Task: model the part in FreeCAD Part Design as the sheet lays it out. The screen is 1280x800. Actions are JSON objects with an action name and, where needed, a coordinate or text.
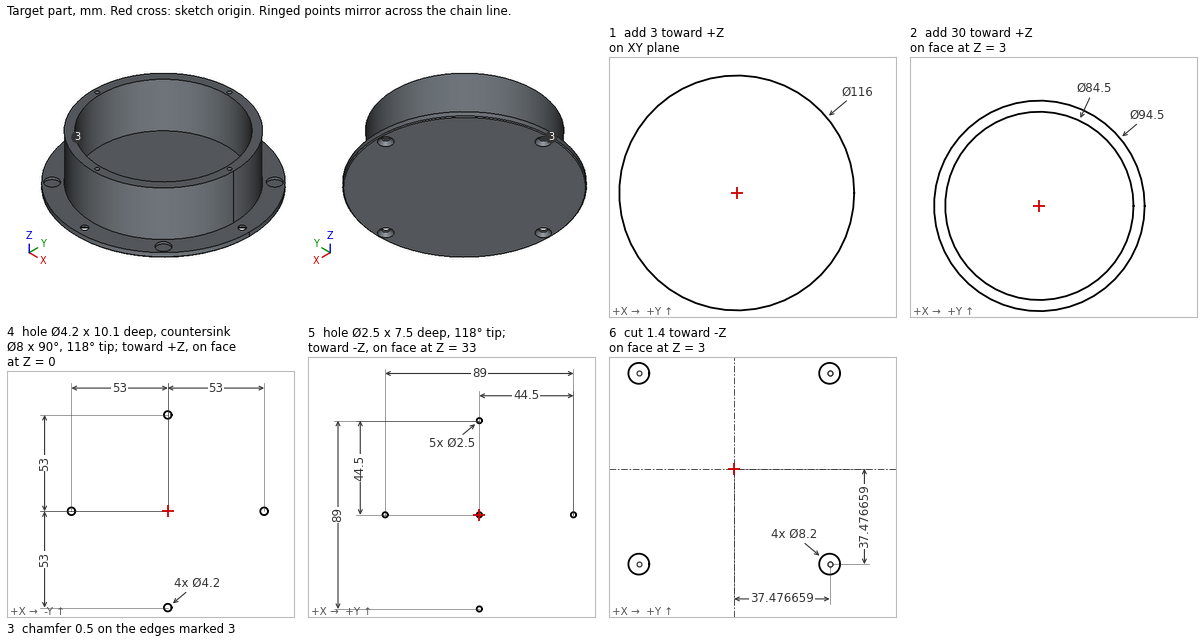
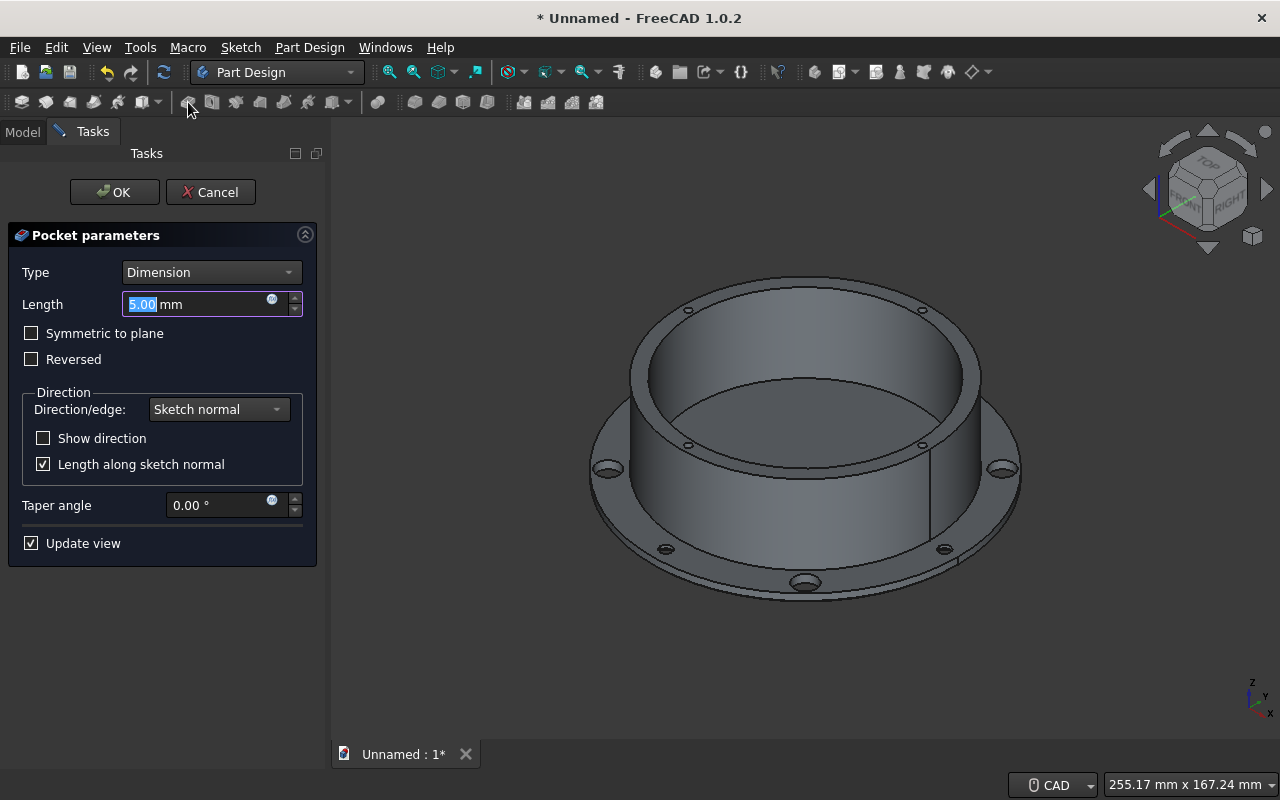
{"action": "type", "text": "1.4"}
{"action": "key", "text": "Tab"}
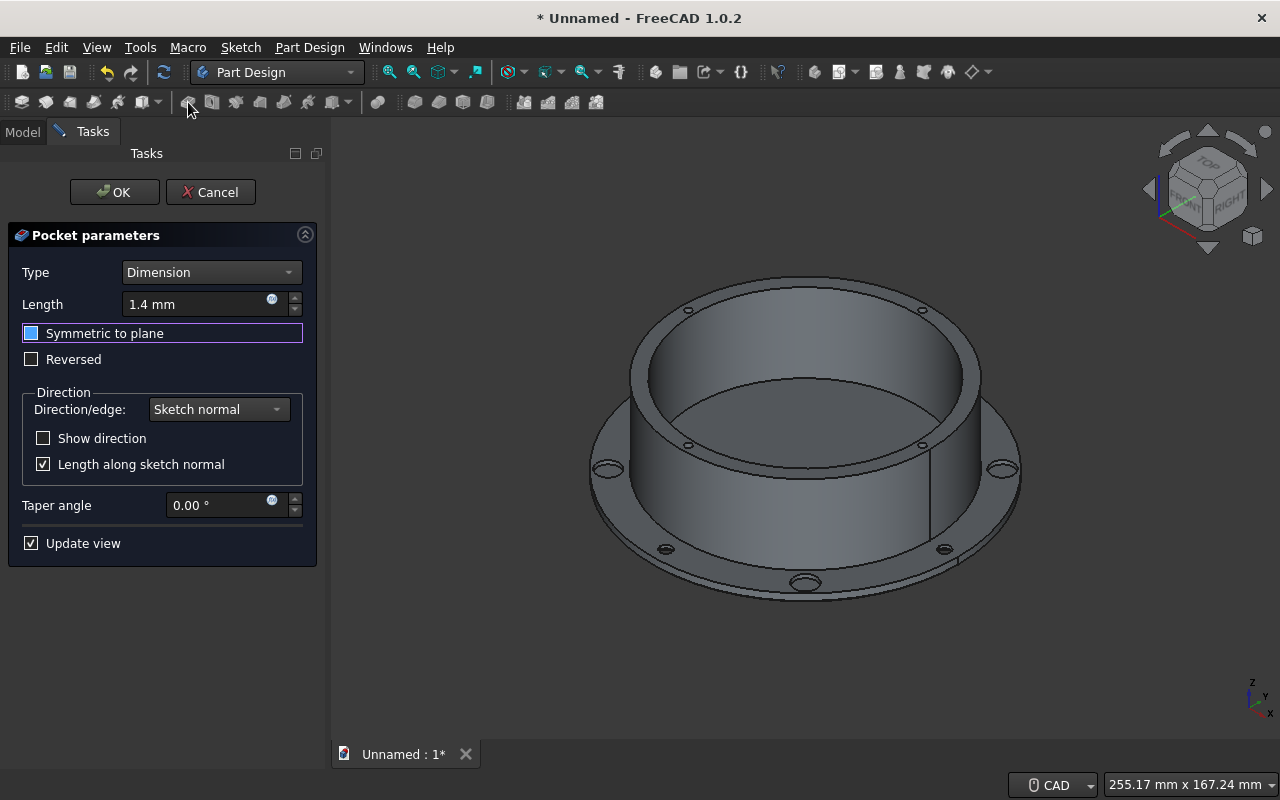
{"action": "left_click", "coordinate": [115, 192]}